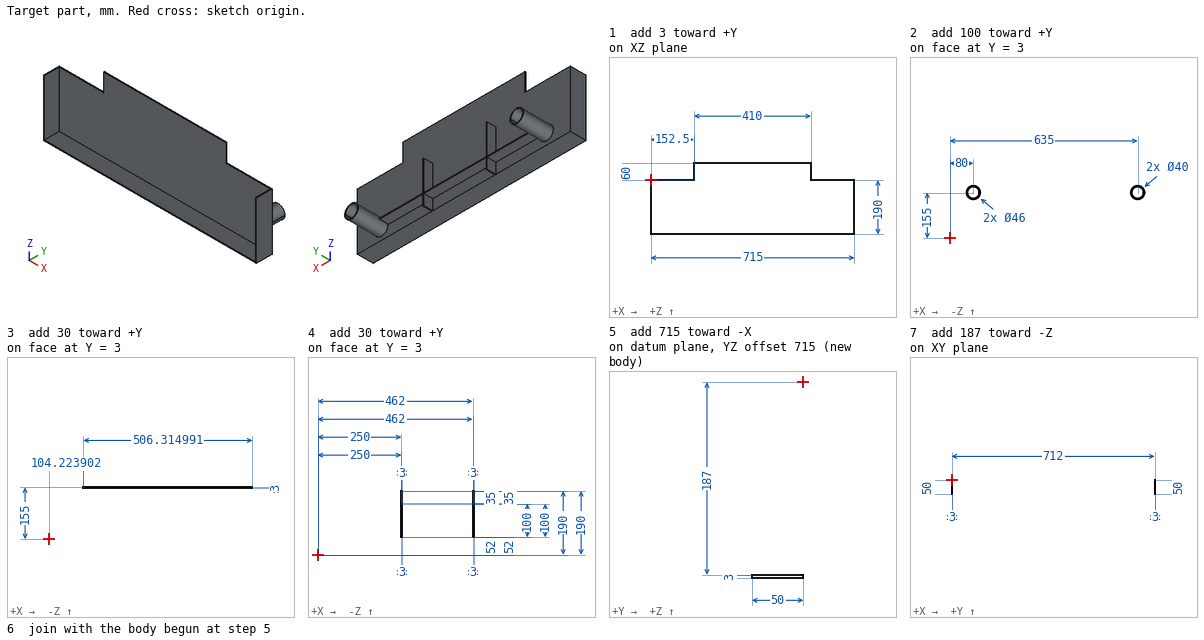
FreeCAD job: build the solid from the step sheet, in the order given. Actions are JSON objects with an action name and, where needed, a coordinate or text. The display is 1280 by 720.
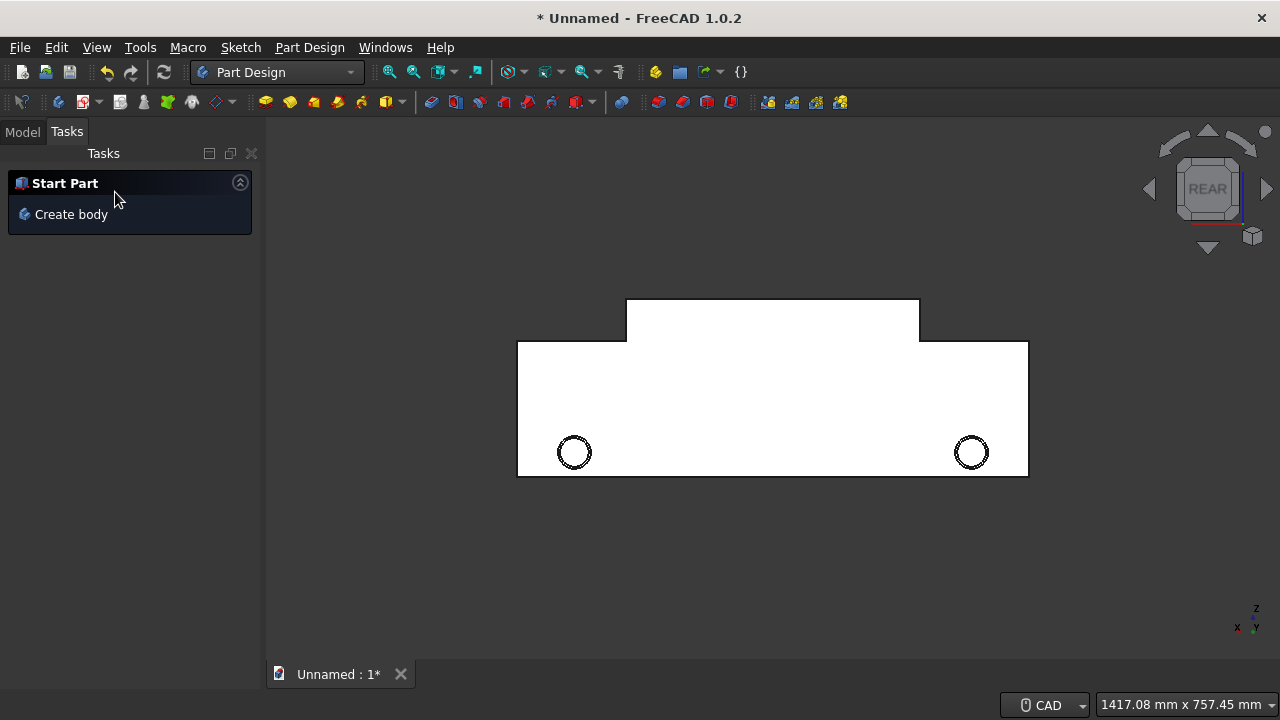
{"action": "left_click", "coordinate": [773, 387]}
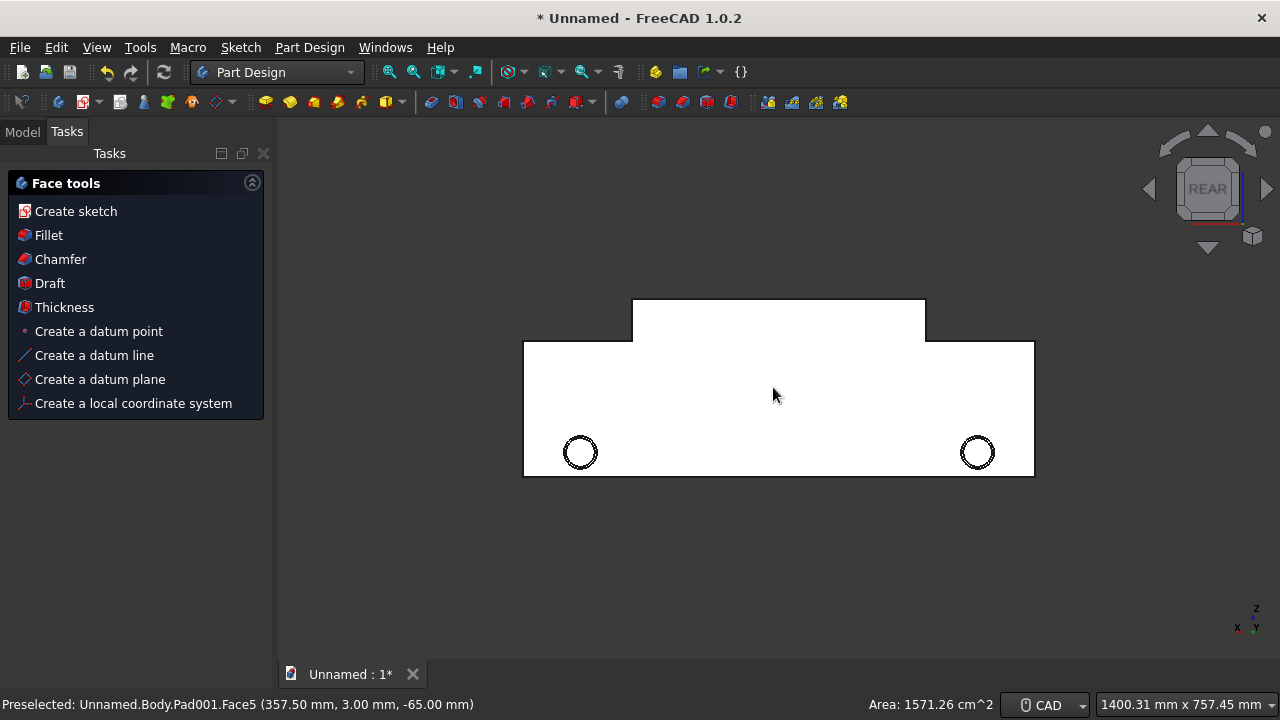
{"action": "left_click", "coordinate": [84, 102]}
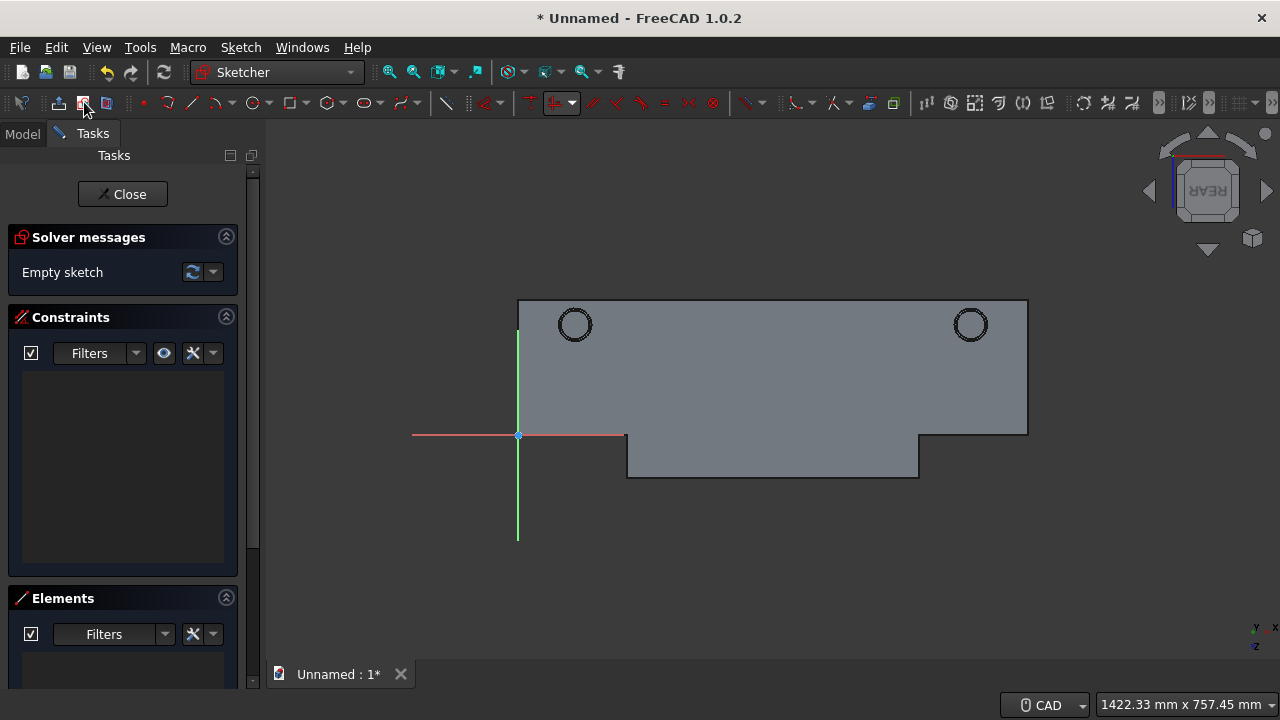
{"action": "key", "text": "q s"}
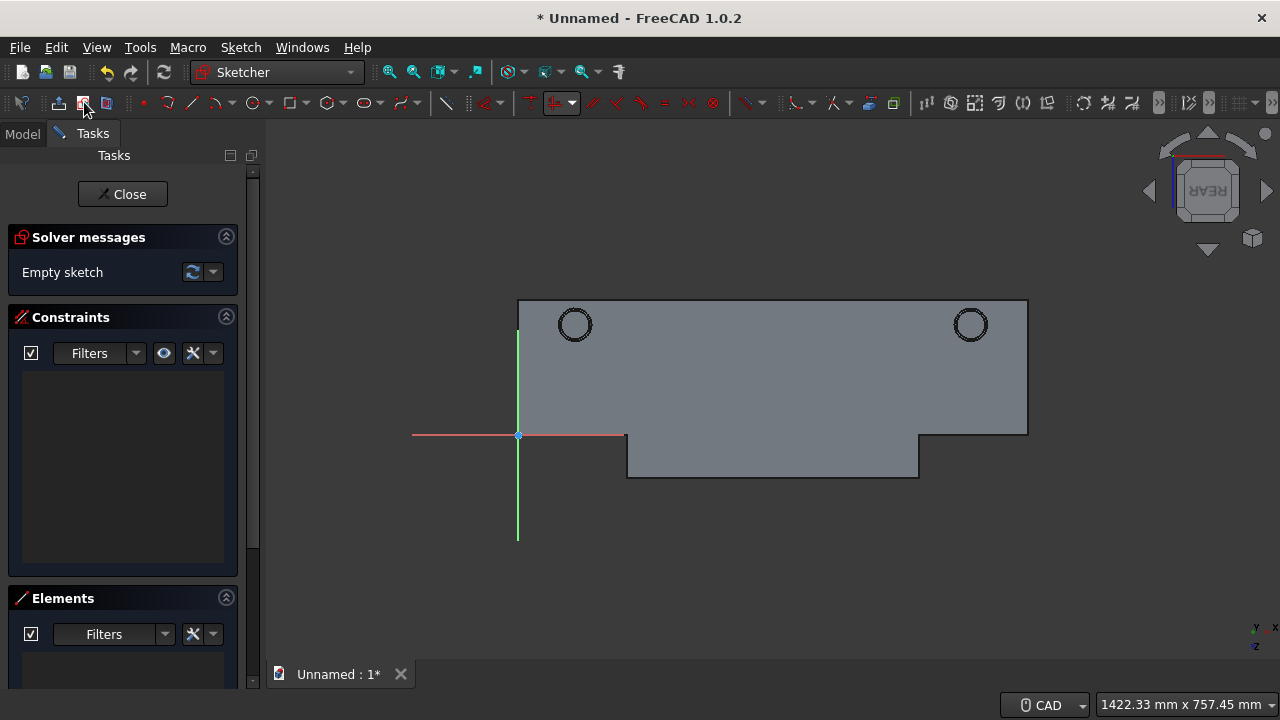
{"action": "left_click", "coordinate": [290, 104]}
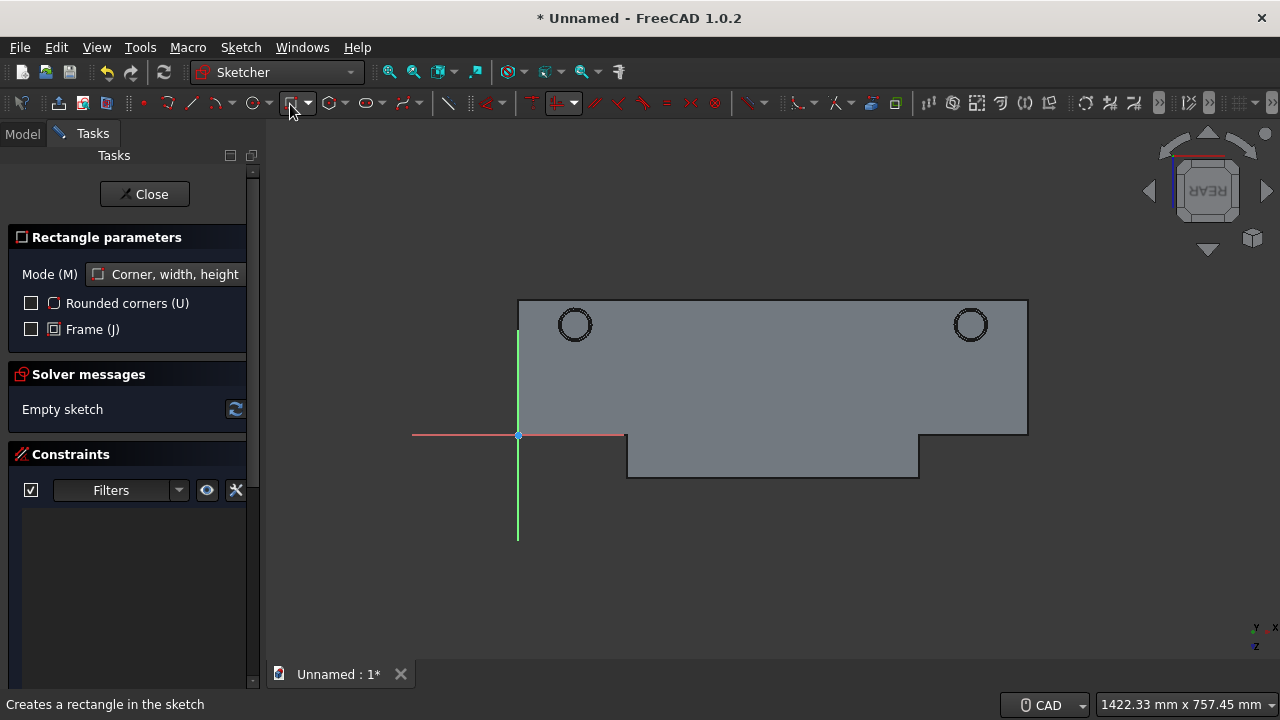
{"action": "scroll", "coordinate": [592, 325], "scroll_direction": "up", "scroll_amount": 11}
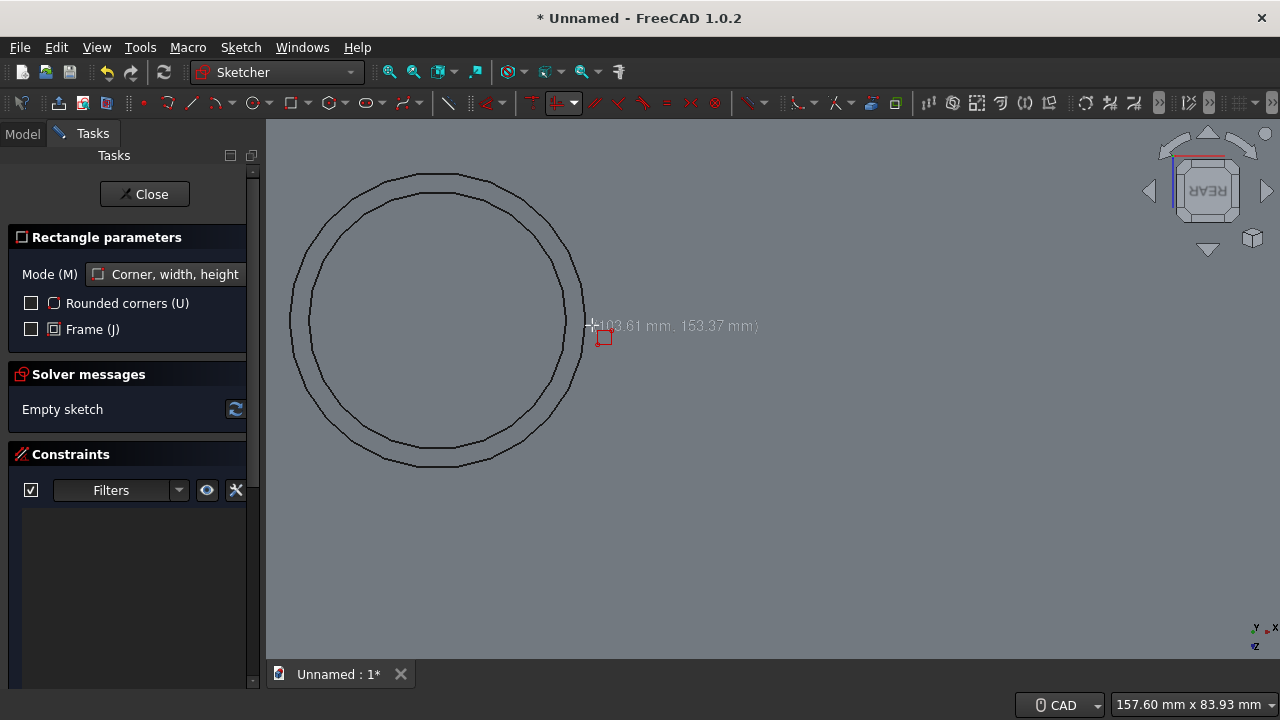
{"action": "scroll", "coordinate": [519, 322], "scroll_direction": "down", "scroll_amount": 10}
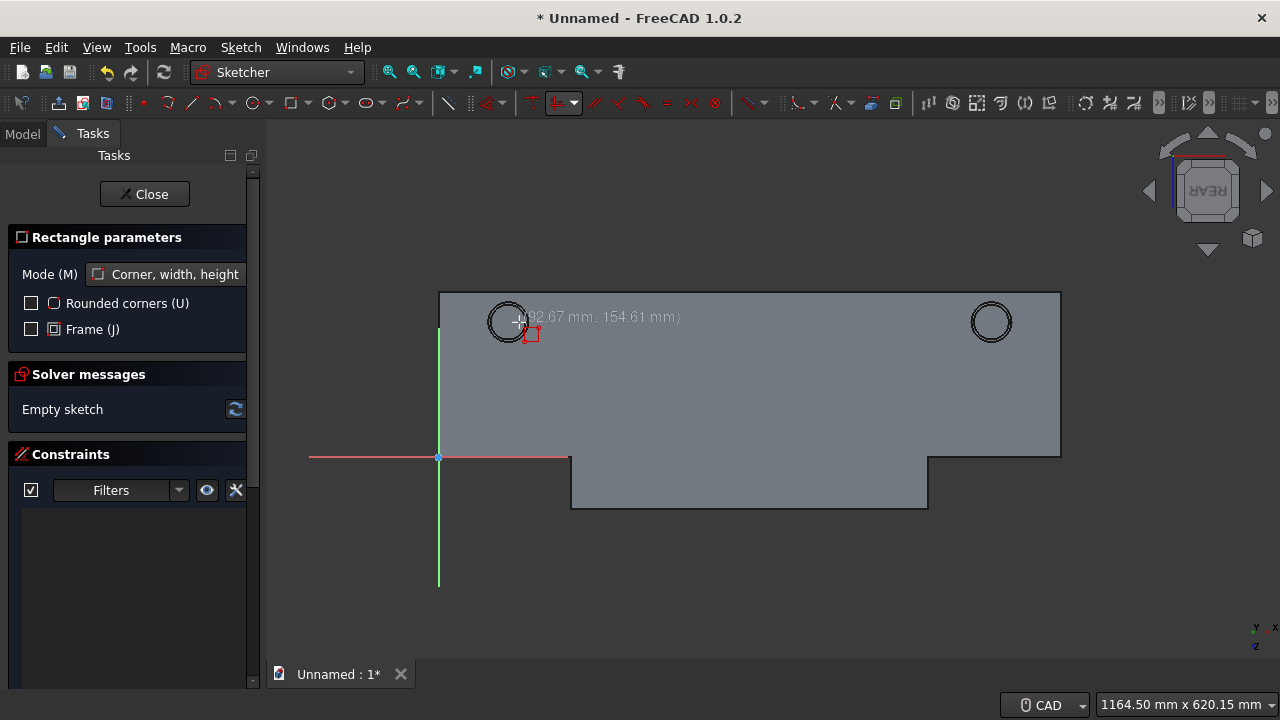
{"action": "left_click", "coordinate": [529, 322]}
{"action": "mouse_move", "coordinate": [970, 325]}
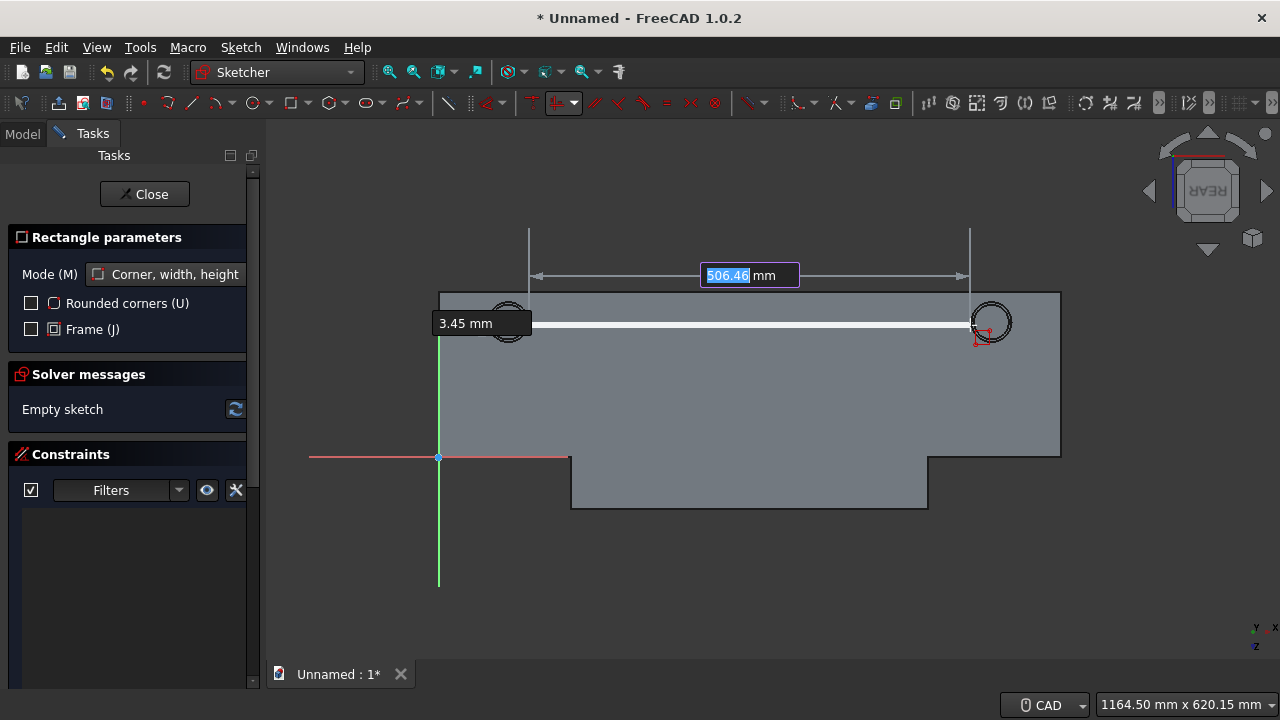
{"action": "type", "text": "506.314991"}
{"action": "key", "text": "Tab"}
{"action": "type", "text": "3"}
{"action": "key", "text": "Return"}
{"action": "key", "text": "Escape"}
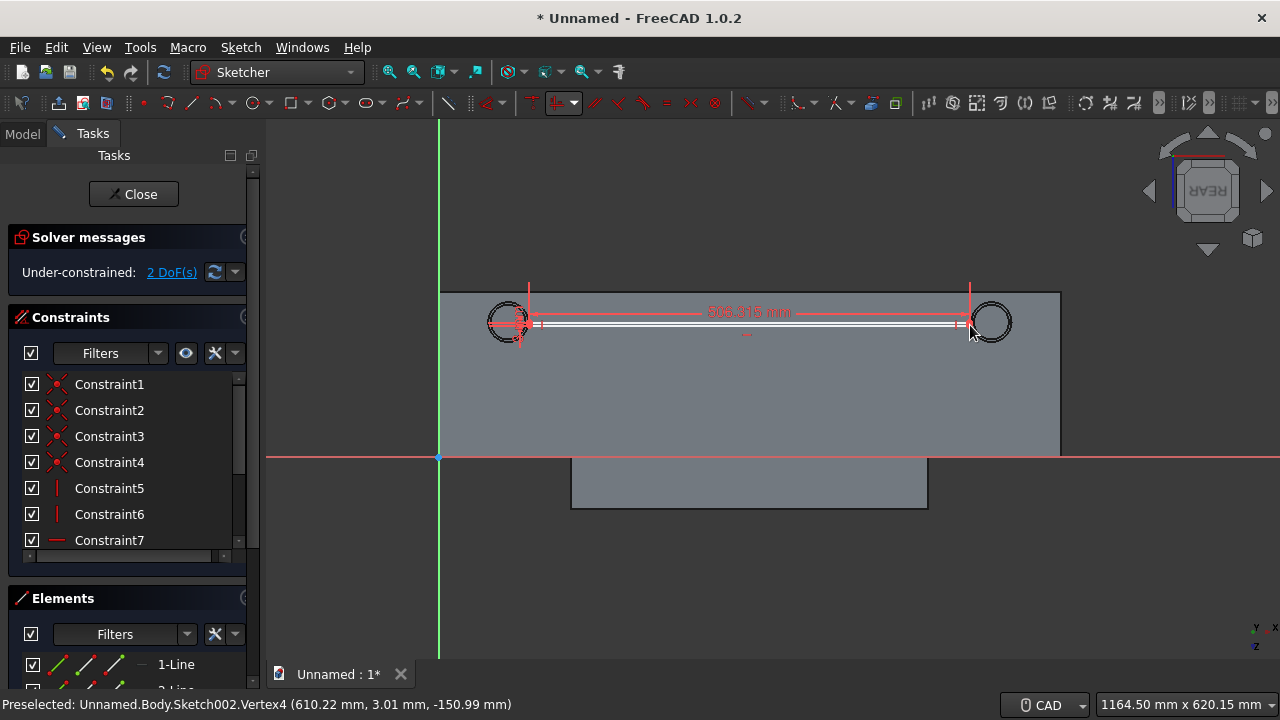
{"action": "left_click", "coordinate": [486, 104]}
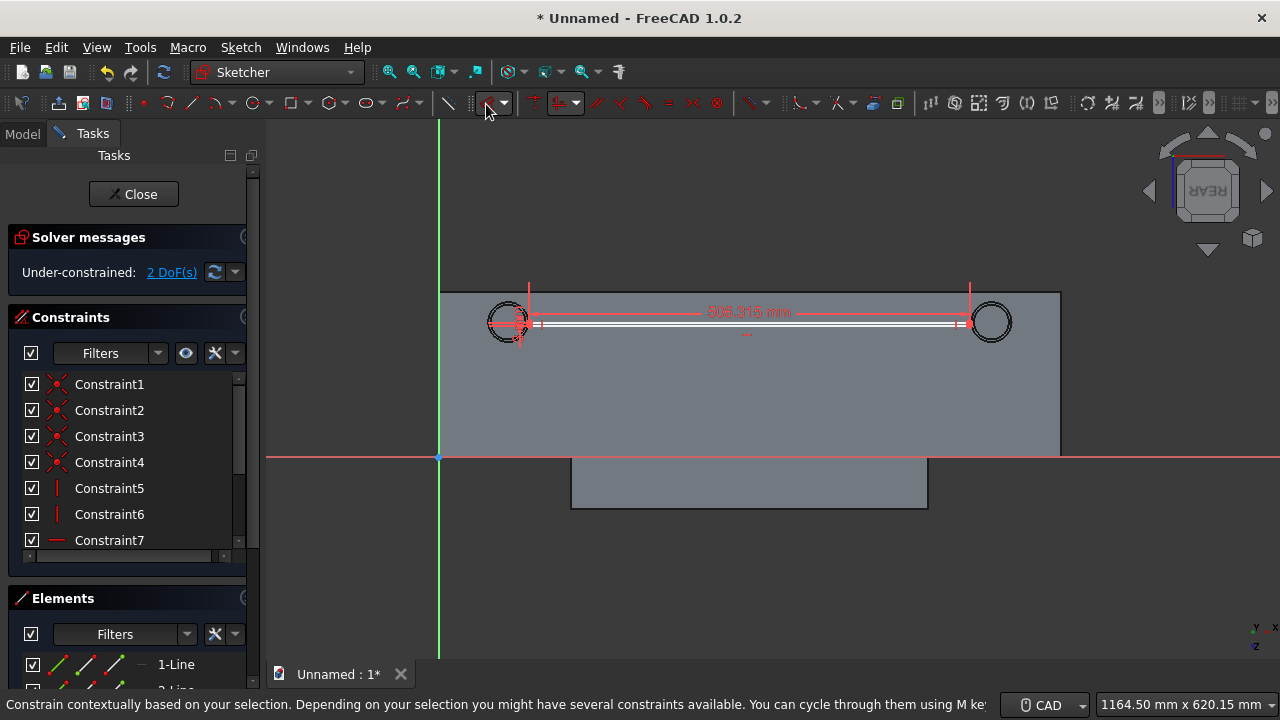
{"action": "scroll", "coordinate": [529, 323], "scroll_direction": "up", "scroll_amount": 8}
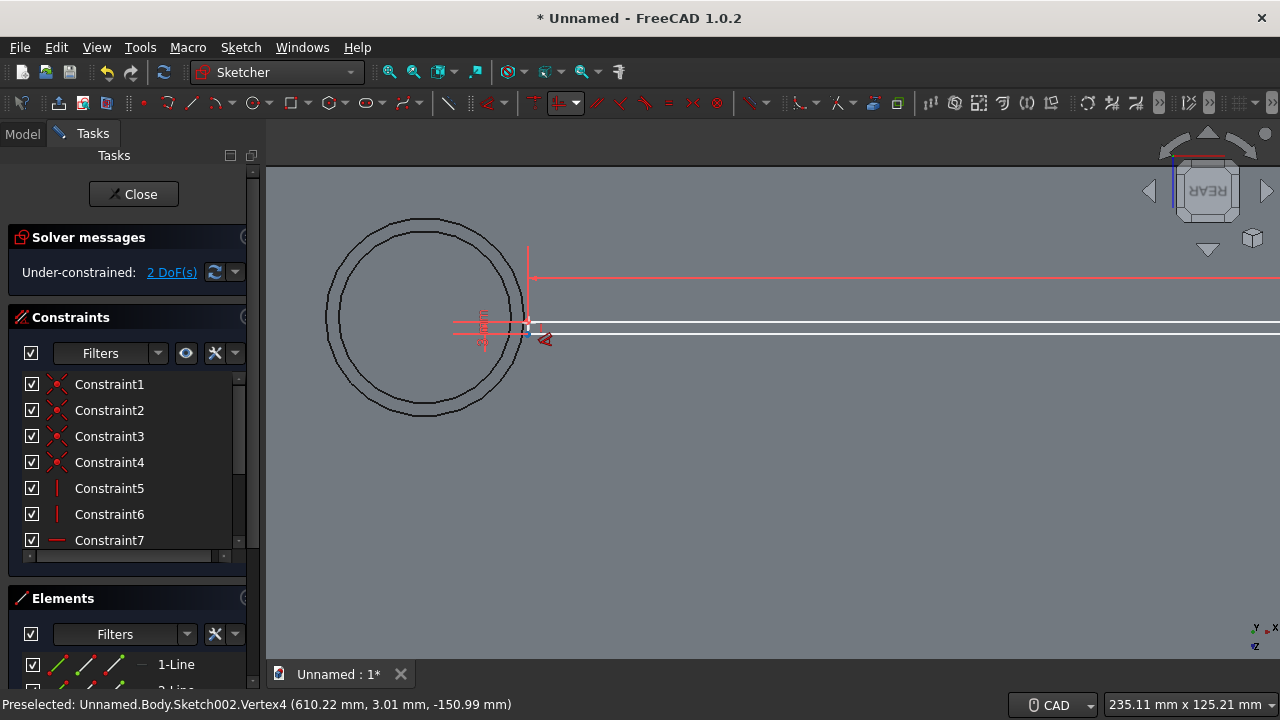
{"action": "left_click", "coordinate": [528, 322]}
{"action": "left_click", "coordinate": [562, 476]}